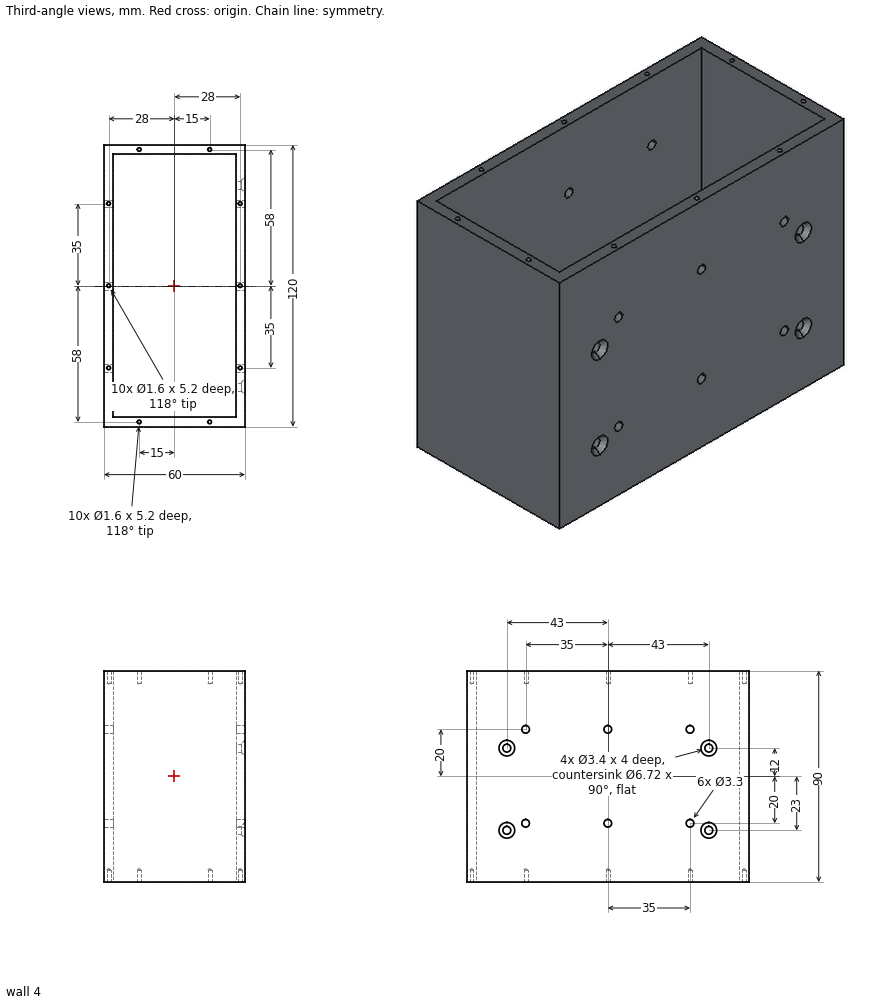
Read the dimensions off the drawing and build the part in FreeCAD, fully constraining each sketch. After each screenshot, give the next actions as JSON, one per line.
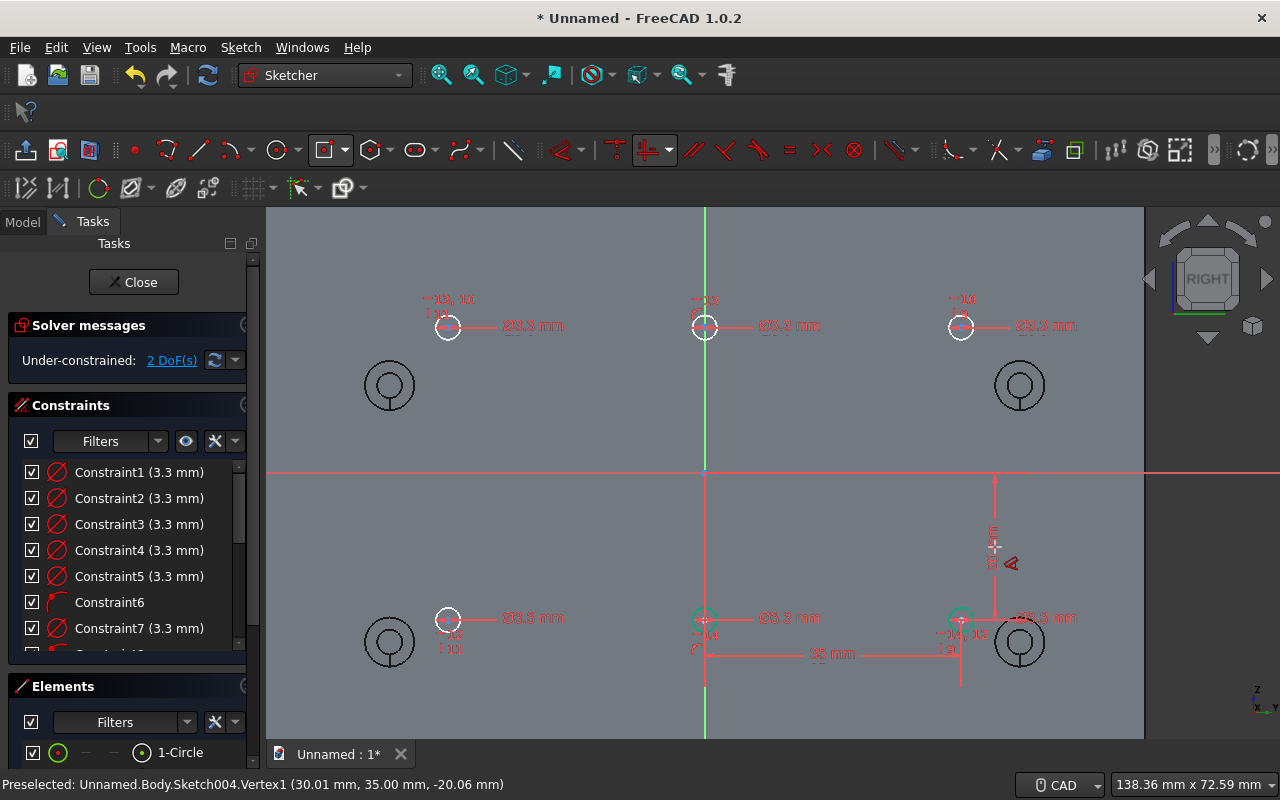
{"action": "left_click", "coordinate": [448, 328]}
{"action": "left_click", "coordinate": [576, 294]}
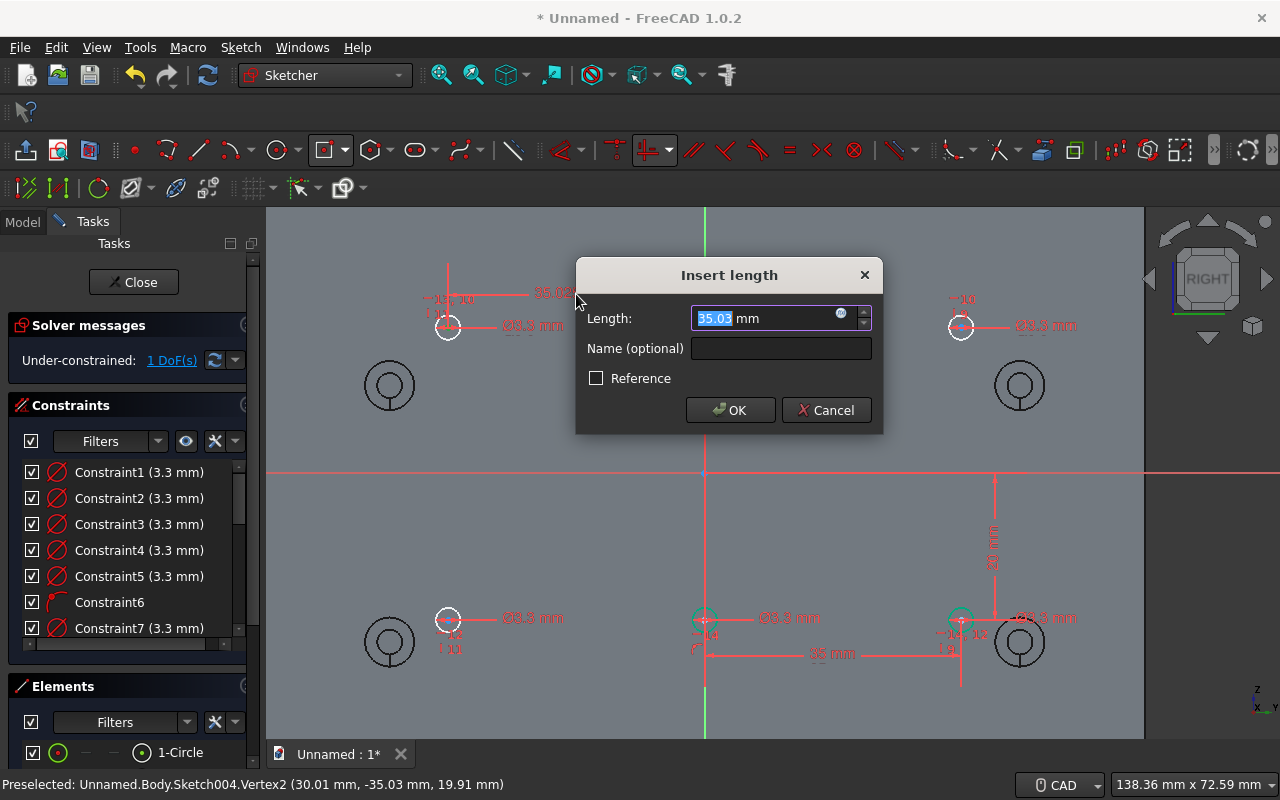
{"action": "type", "text": "35"}
{"action": "key", "text": "Return"}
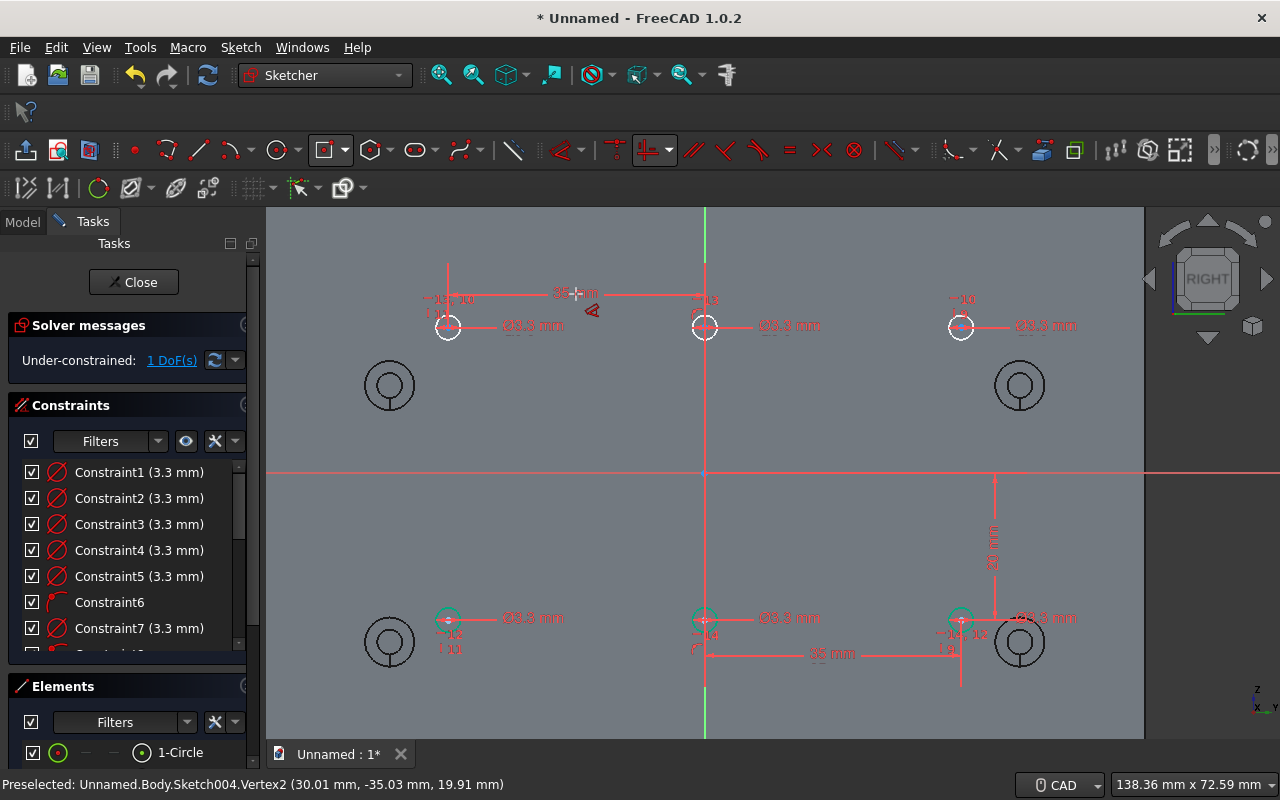
{"action": "left_click", "coordinate": [448, 328]}
{"action": "left_click", "coordinate": [414, 401]}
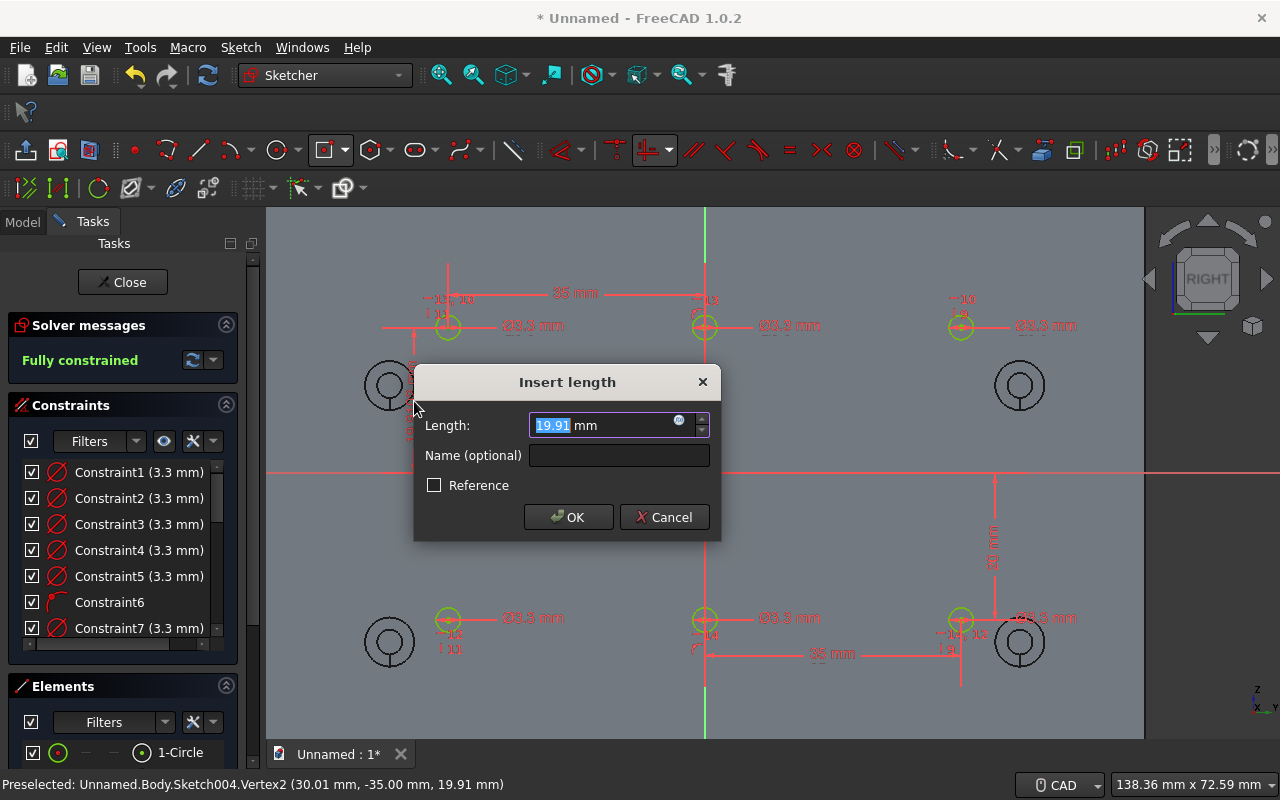
{"action": "type", "text": "20"}
{"action": "key", "text": "Return"}
{"action": "key", "text": "Escape"}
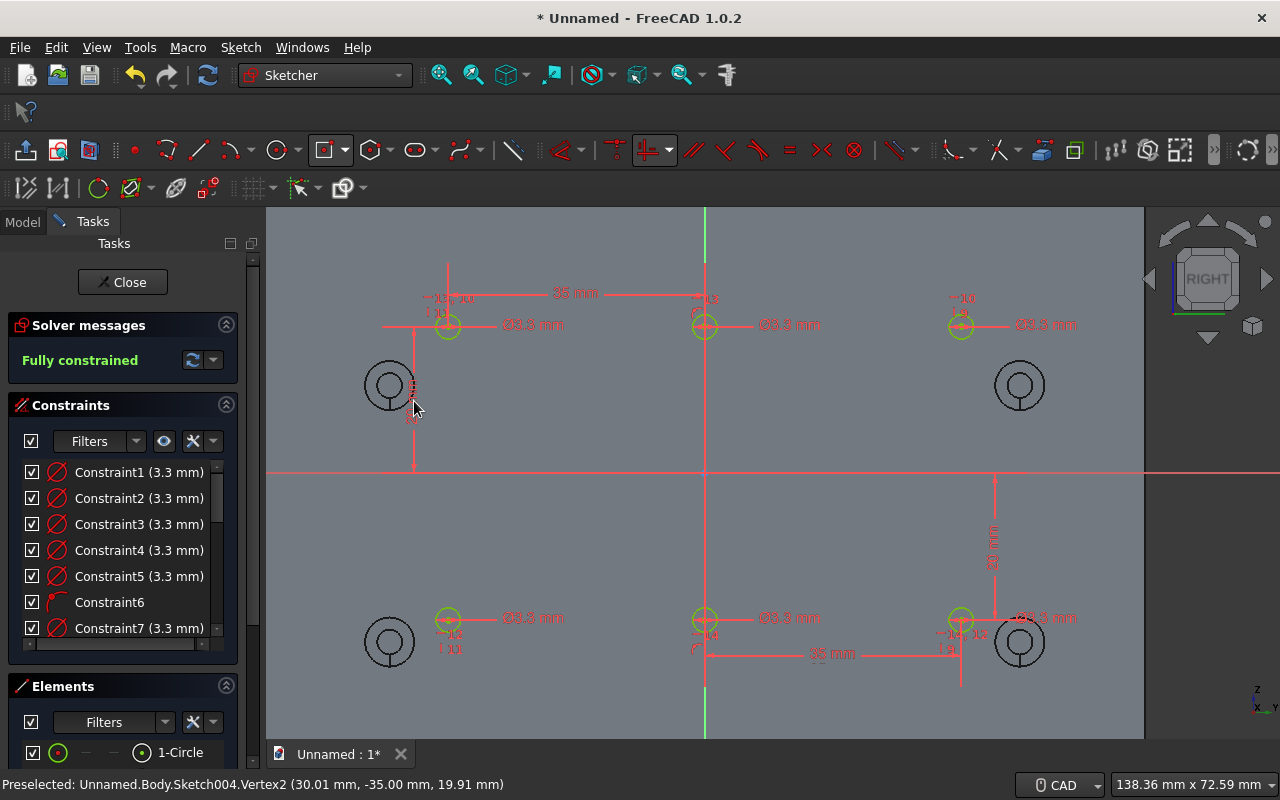
{"action": "left_click", "coordinate": [123, 282]}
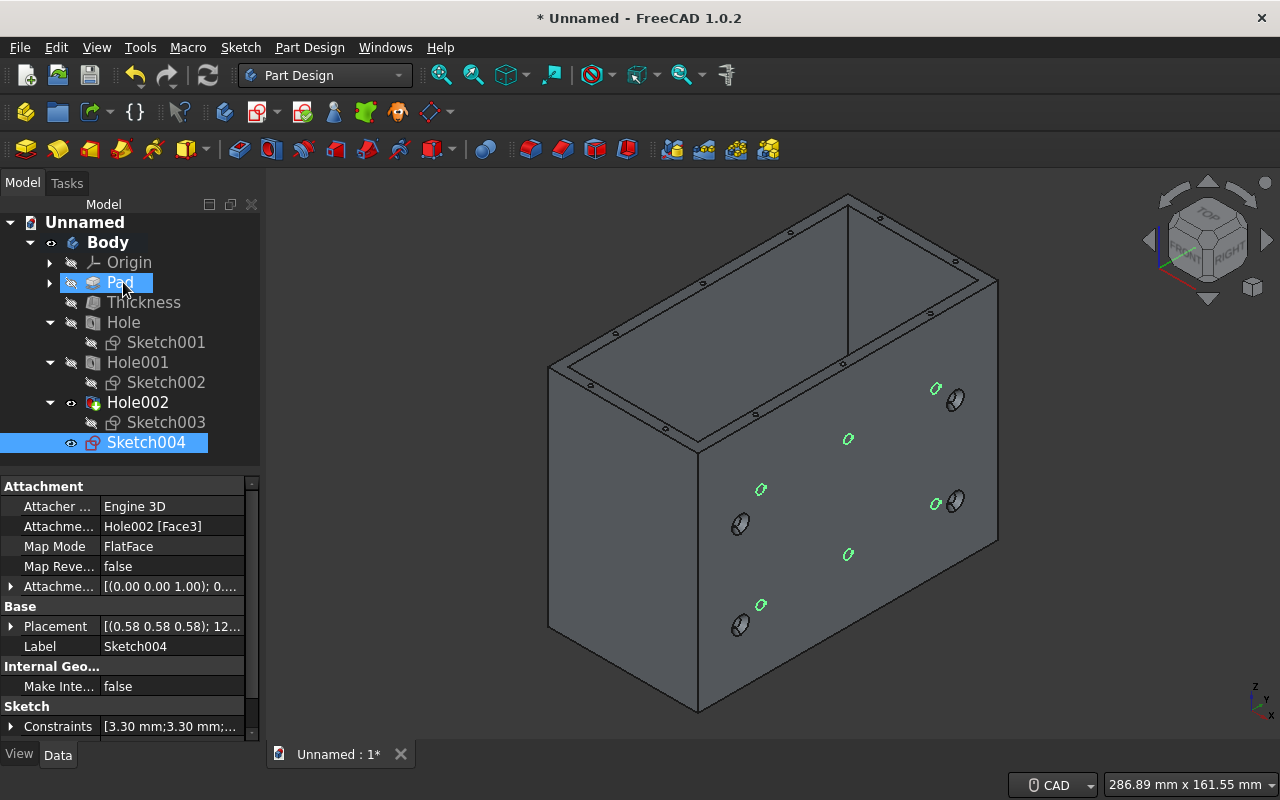
{"action": "left_click", "coordinate": [240, 150]}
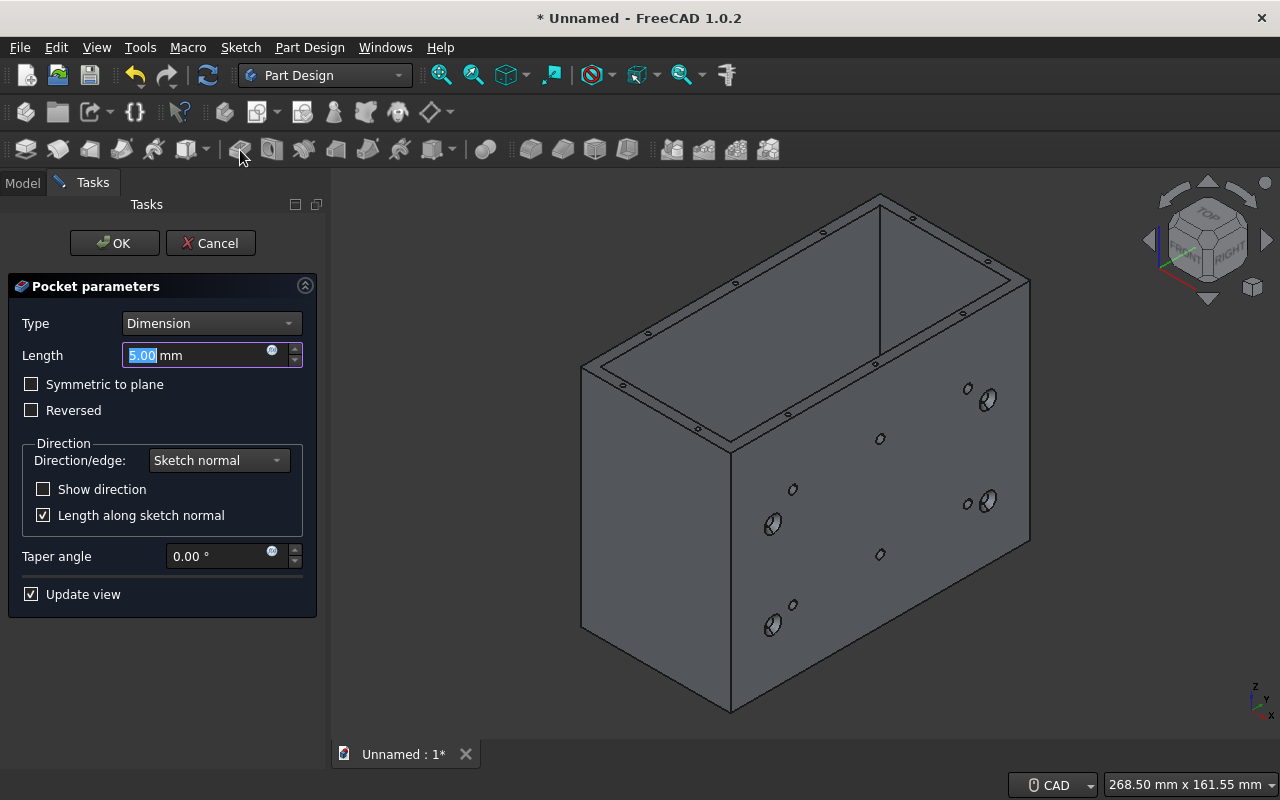
{"action": "left_click", "coordinate": [212, 324]}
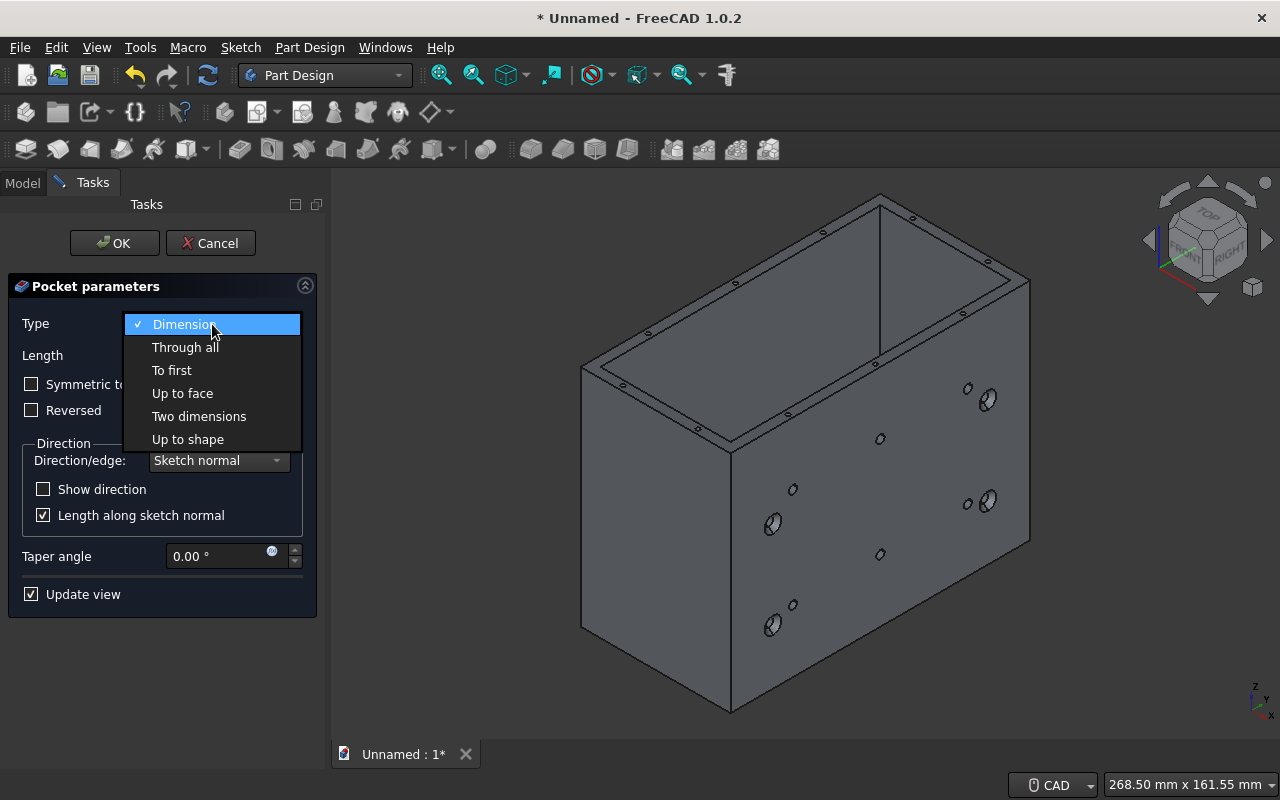
{"action": "left_click", "coordinate": [212, 348]}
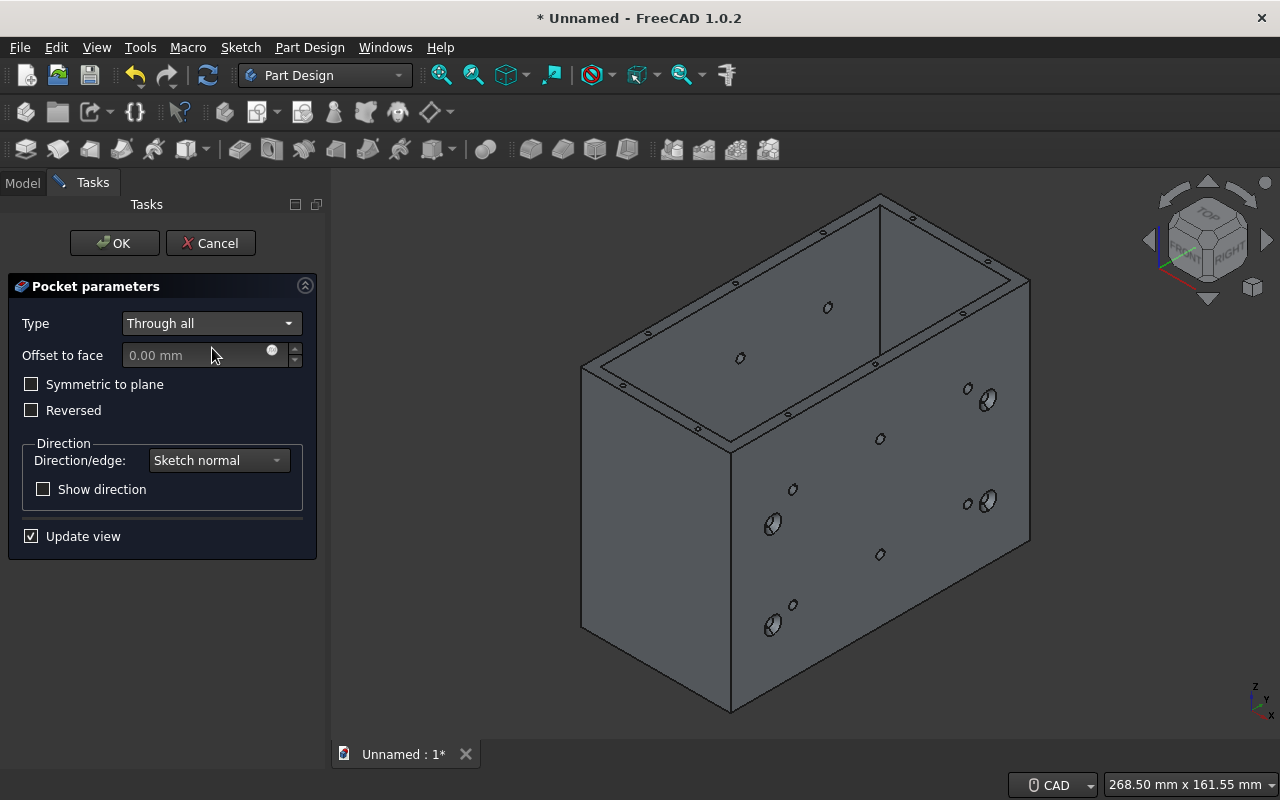
{"action": "left_click", "coordinate": [115, 243]}